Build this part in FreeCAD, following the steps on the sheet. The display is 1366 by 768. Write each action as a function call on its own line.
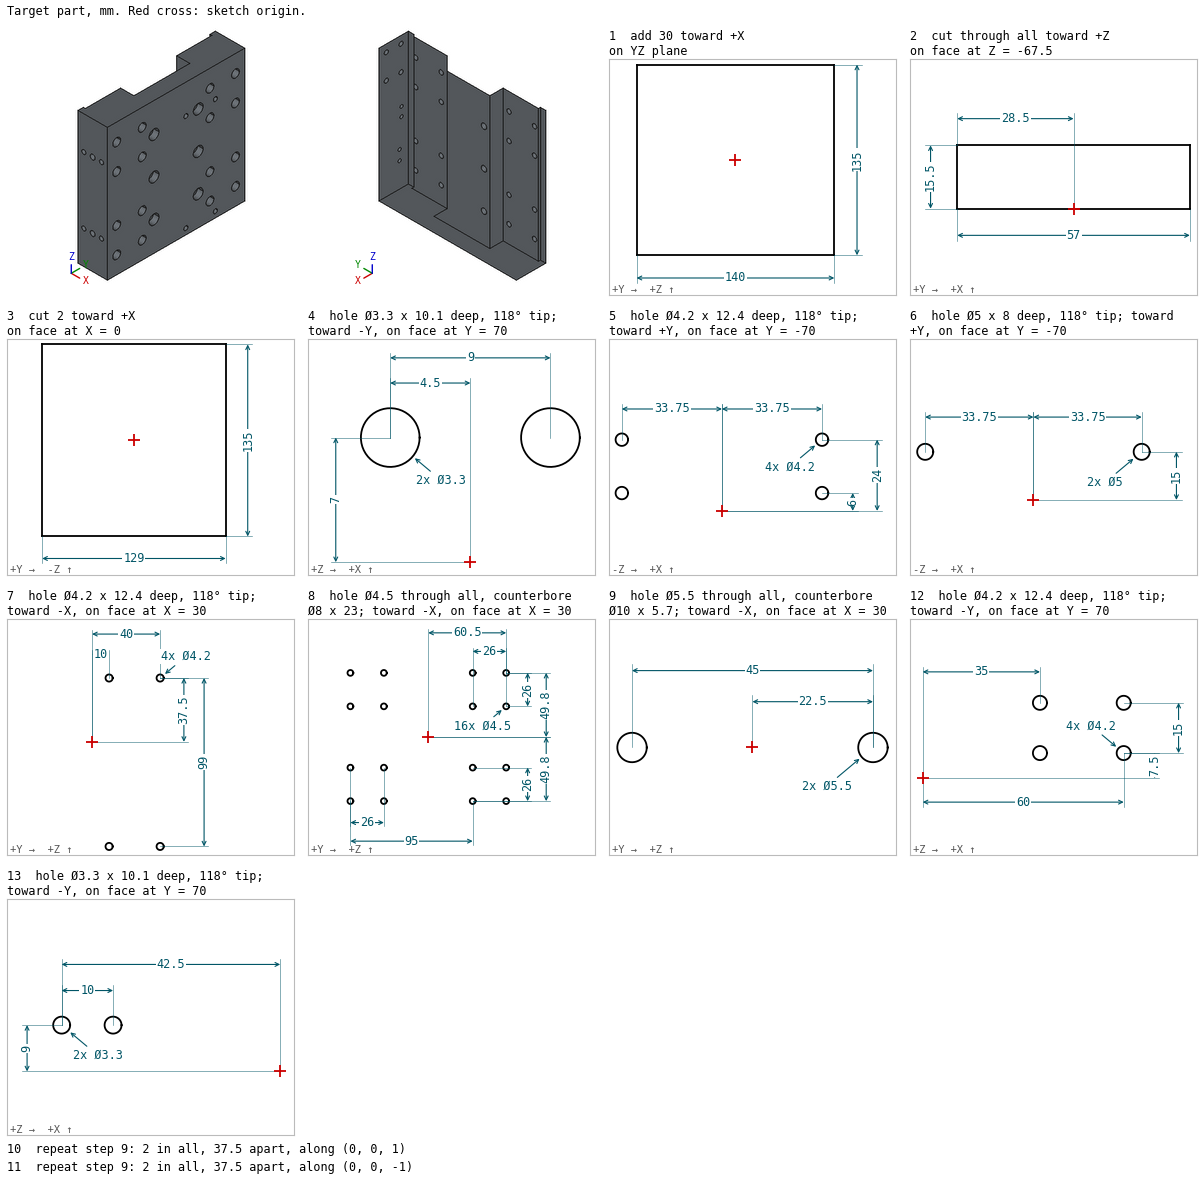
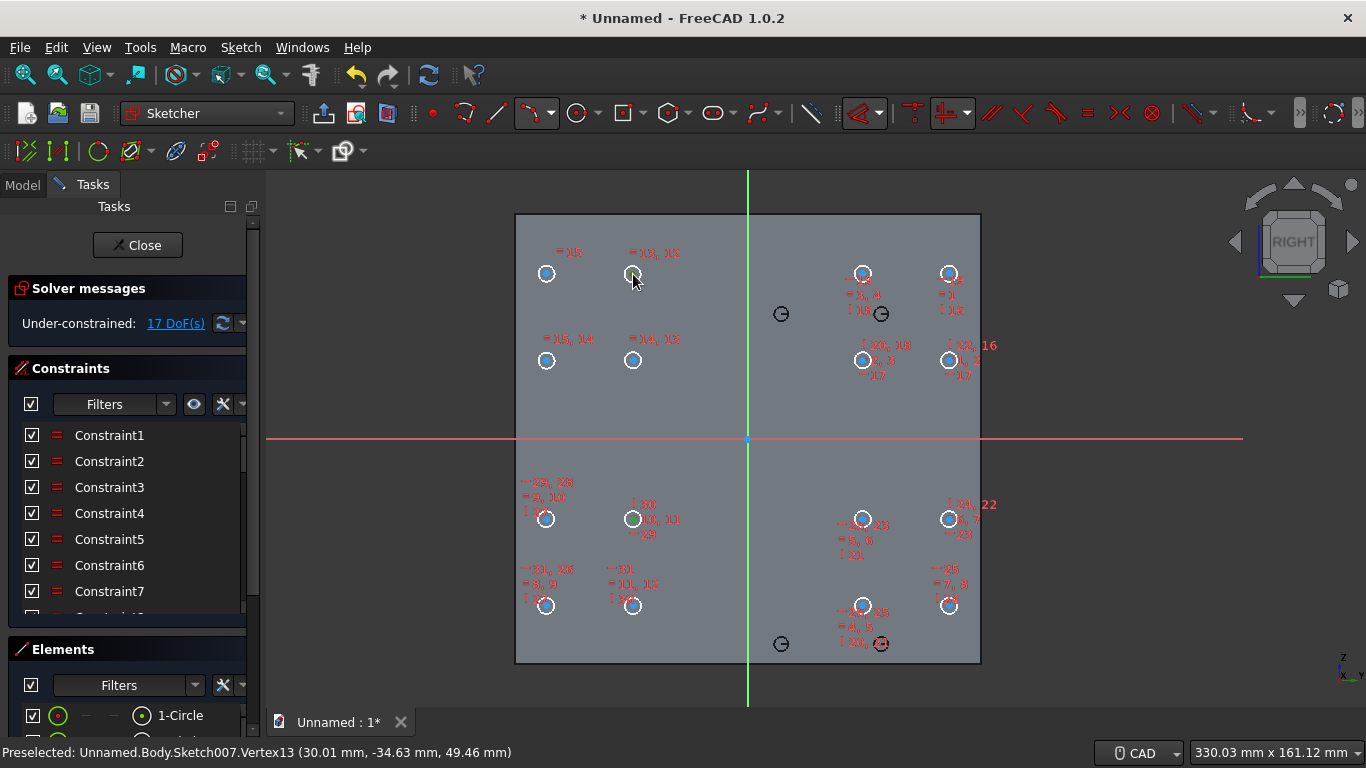
click(970, 114)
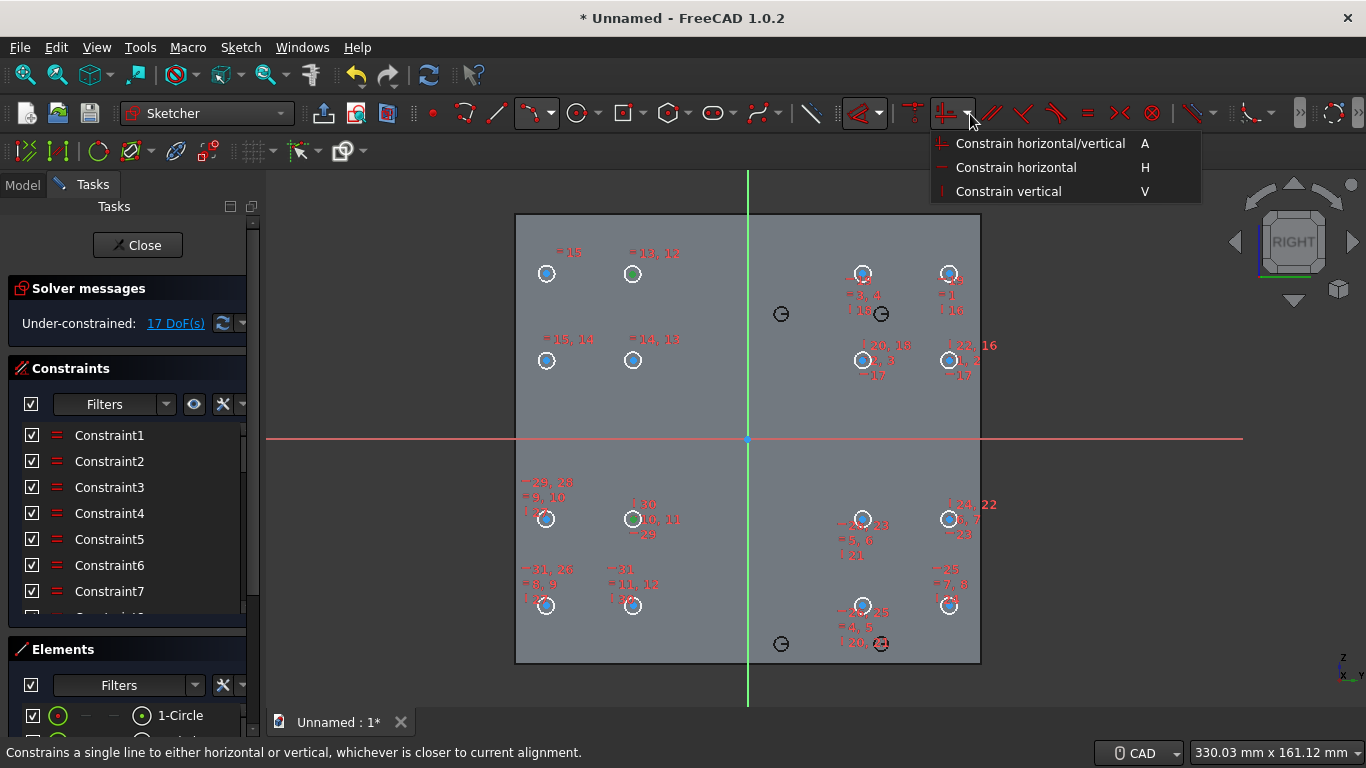
click(1066, 191)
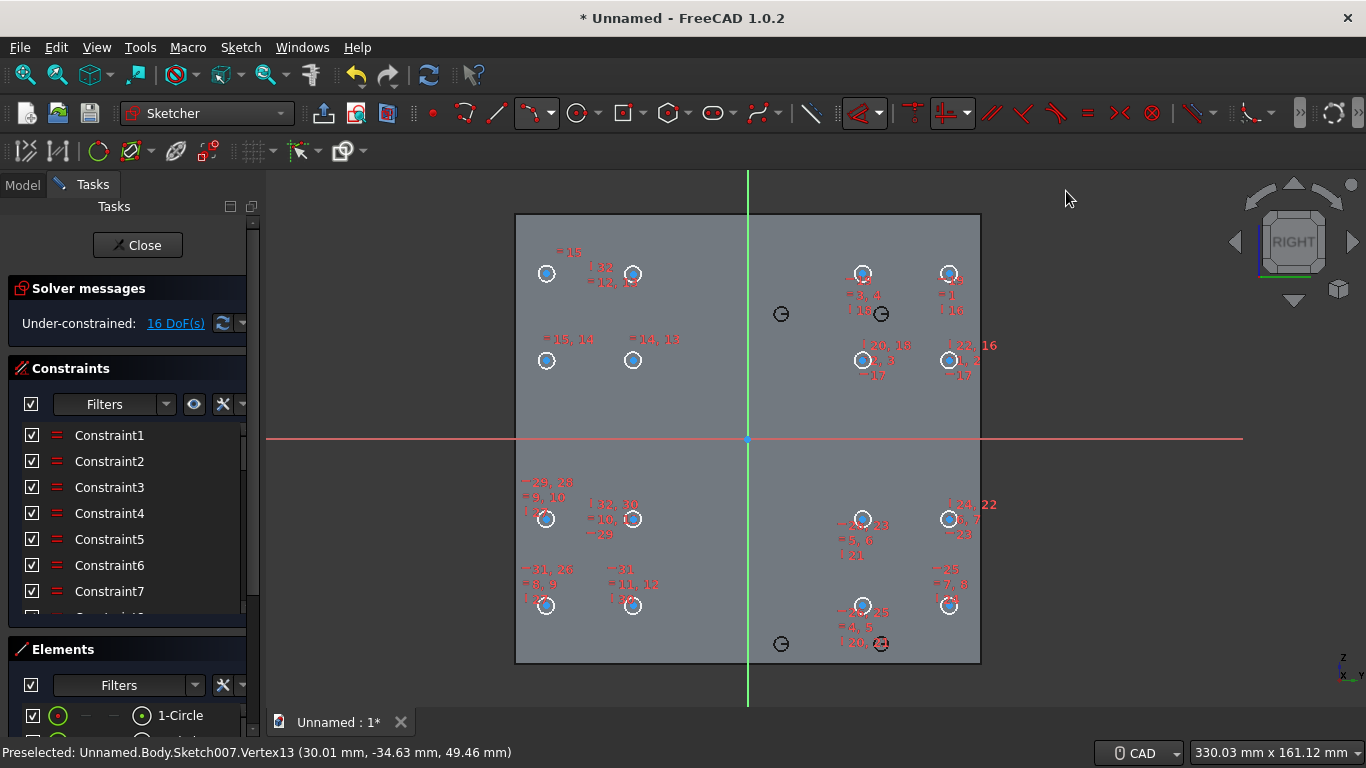
scroll(863, 274, up, 4)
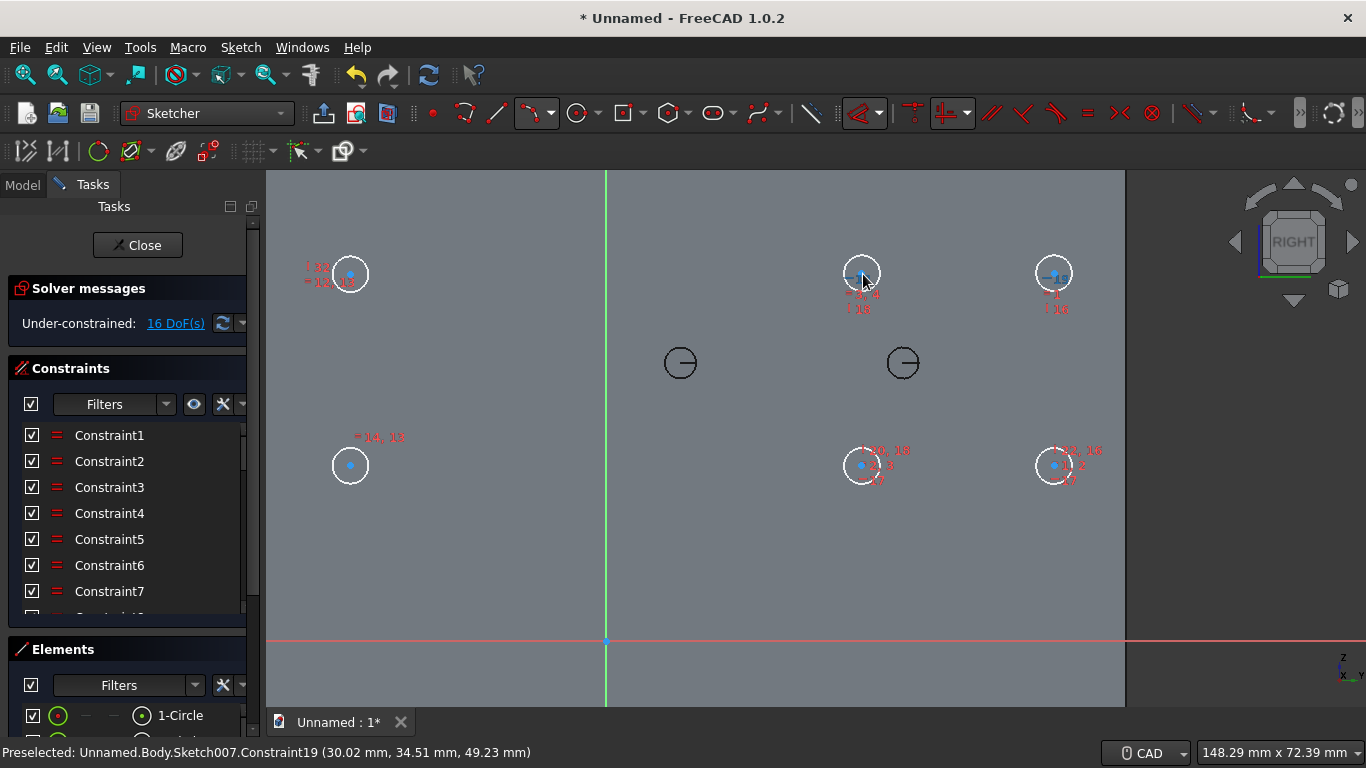
click(860, 271)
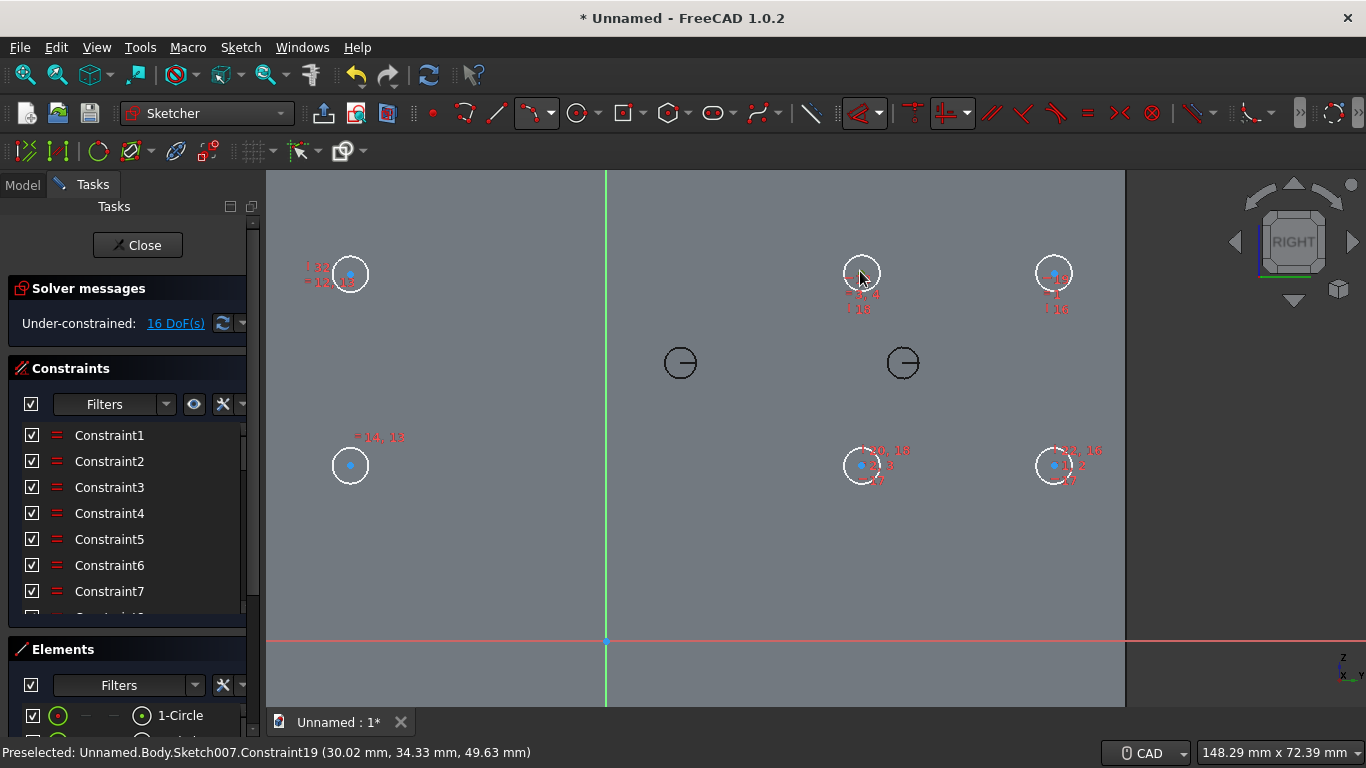
scroll(350, 274, up, 4)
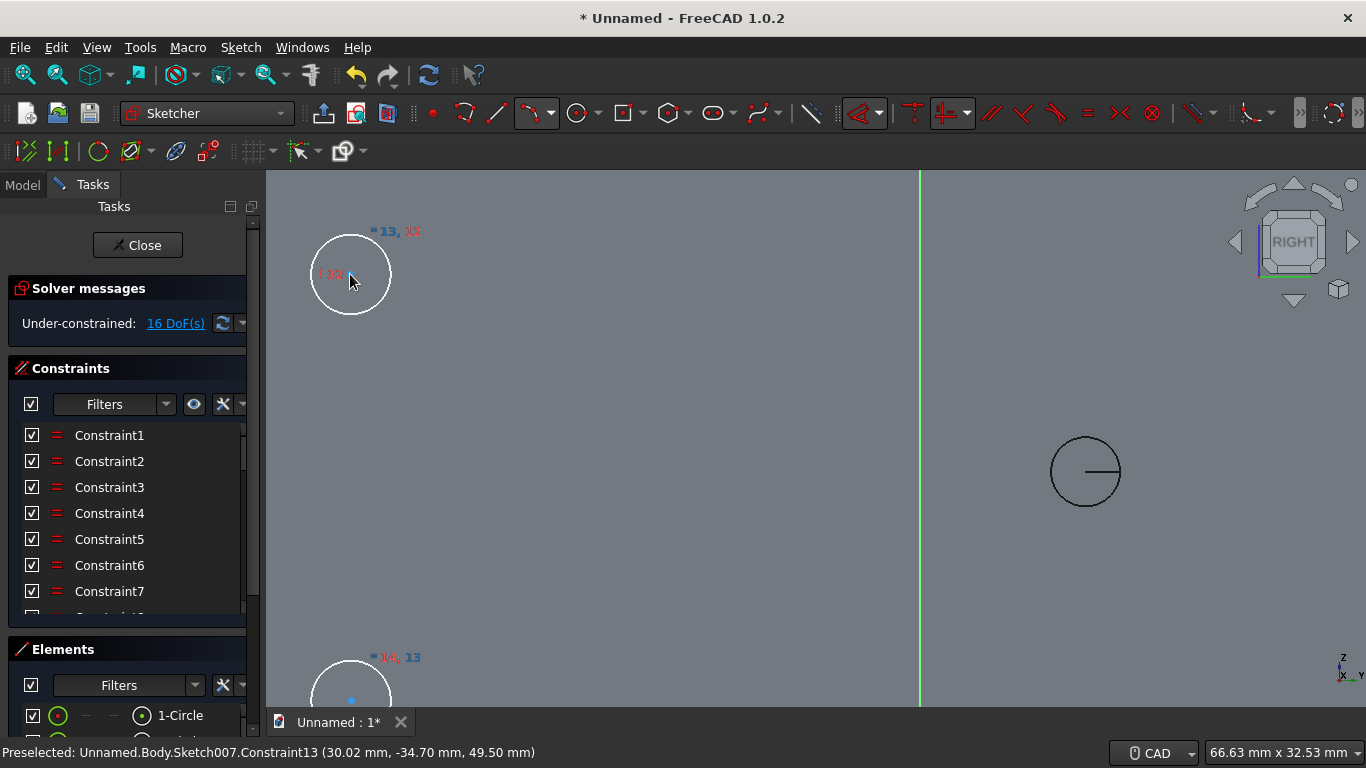
click(351, 274)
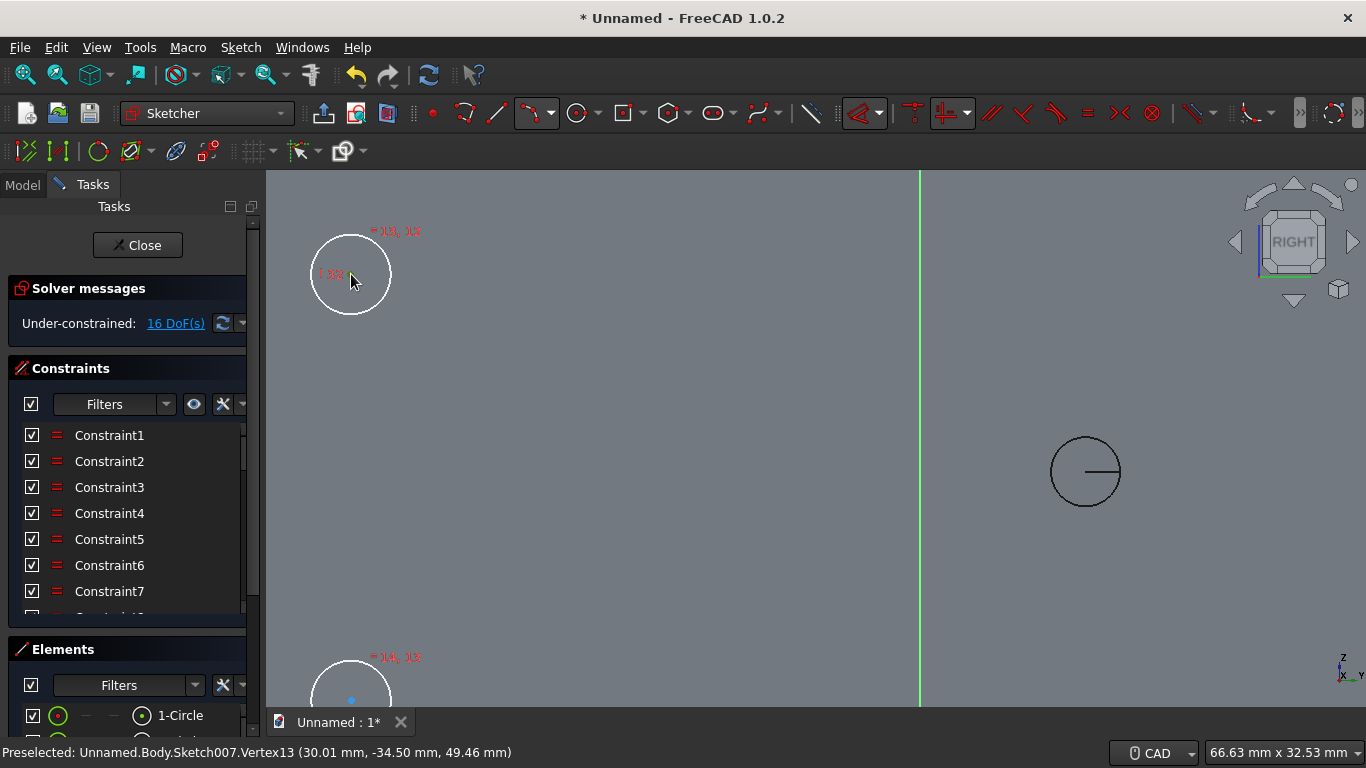
key(h)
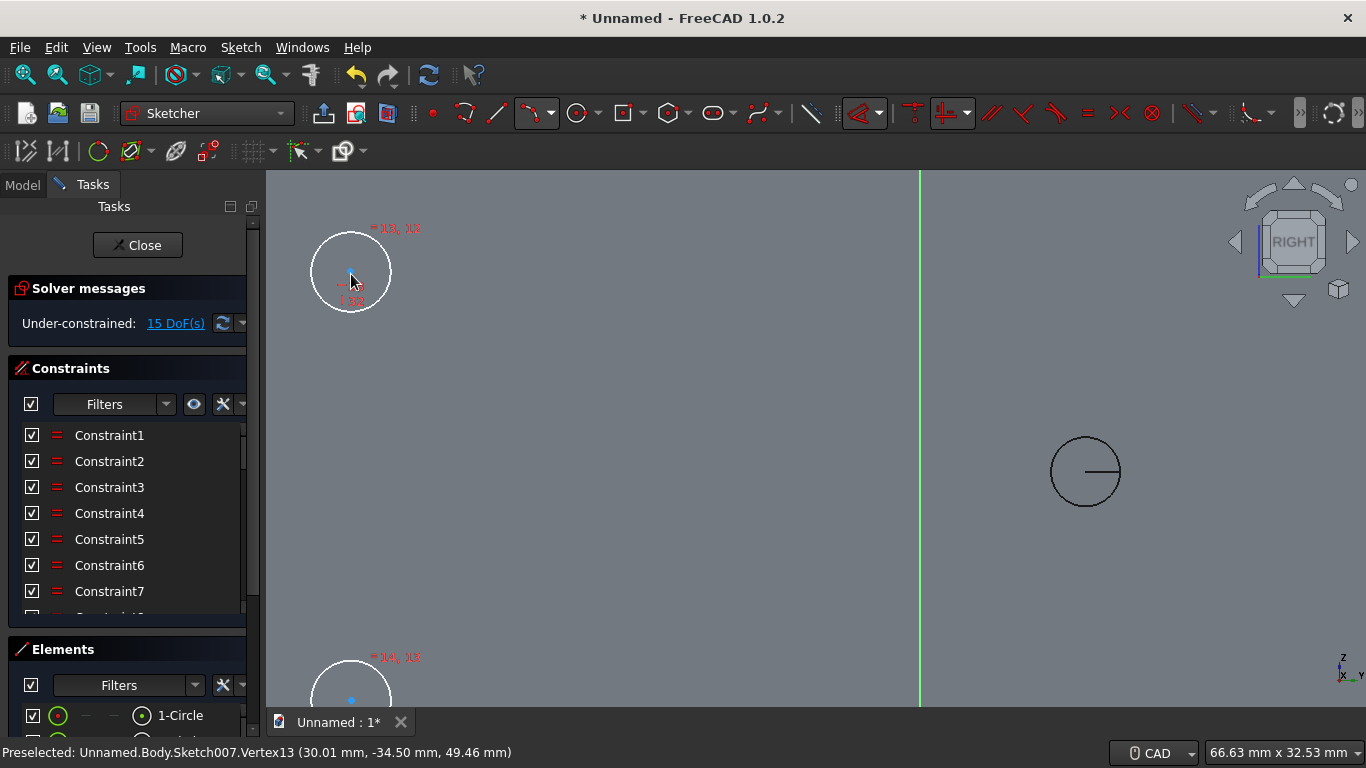
scroll(704, 273, down, 8)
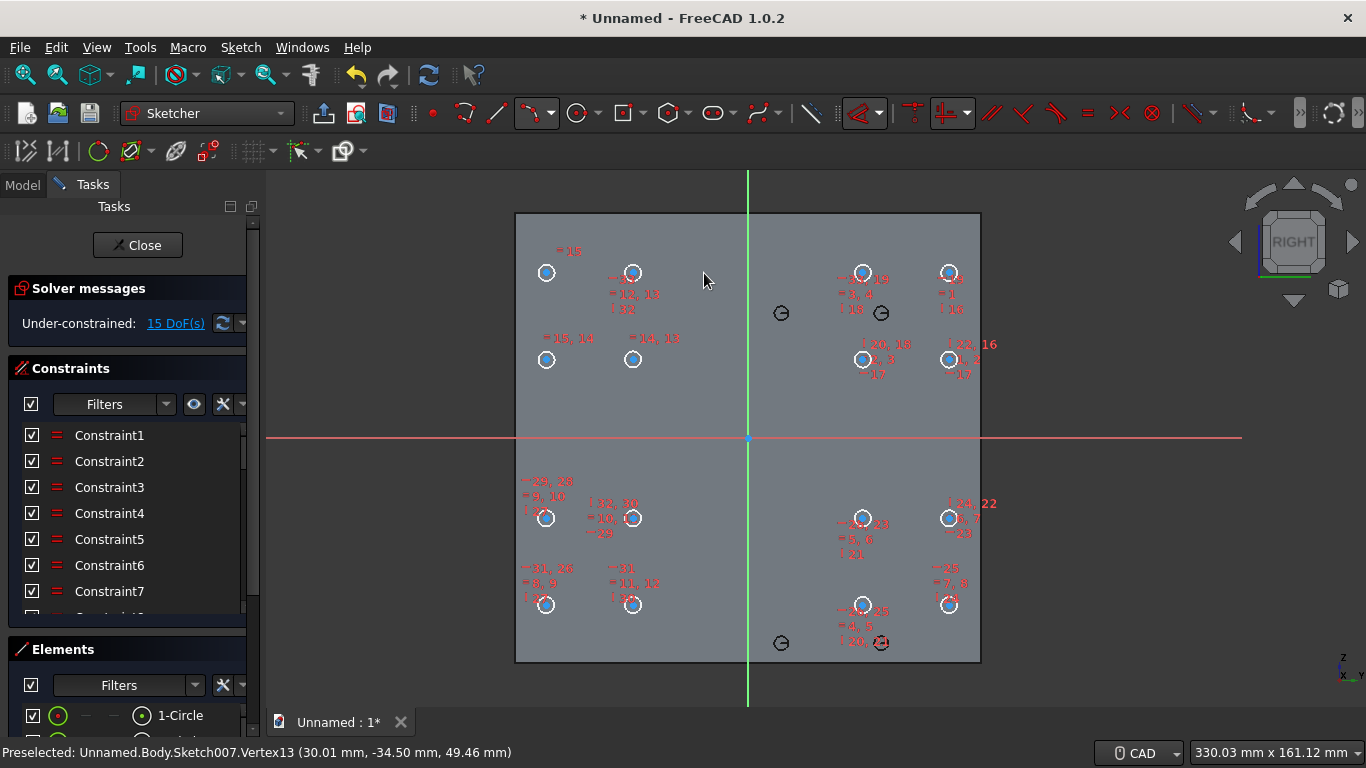
scroll(633, 273, up, 4)